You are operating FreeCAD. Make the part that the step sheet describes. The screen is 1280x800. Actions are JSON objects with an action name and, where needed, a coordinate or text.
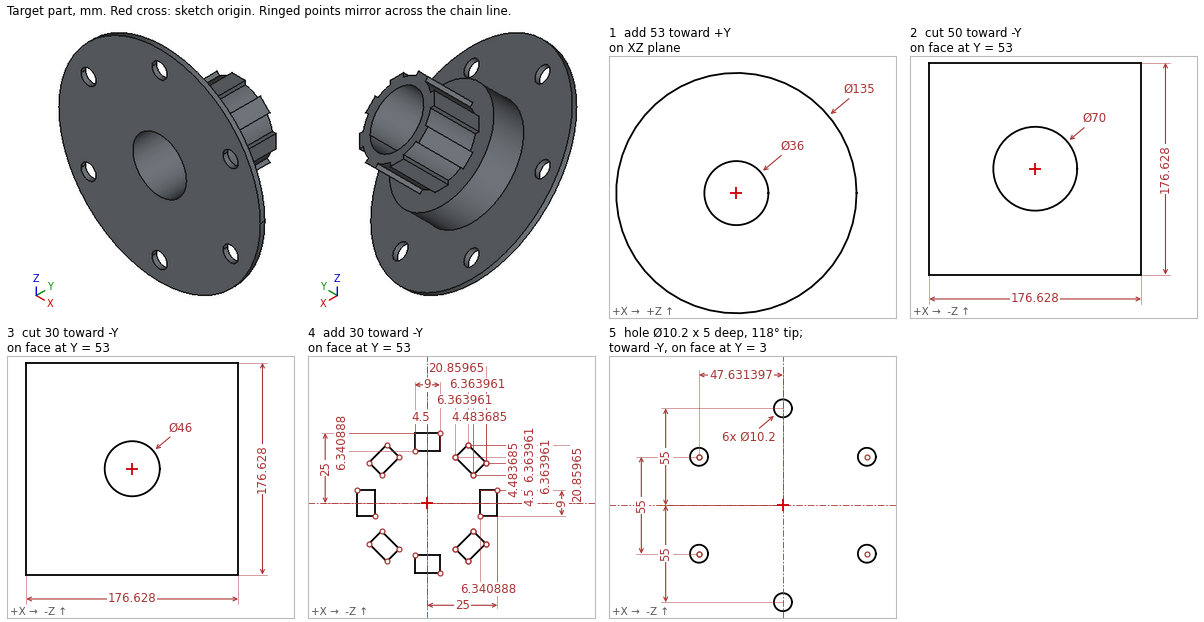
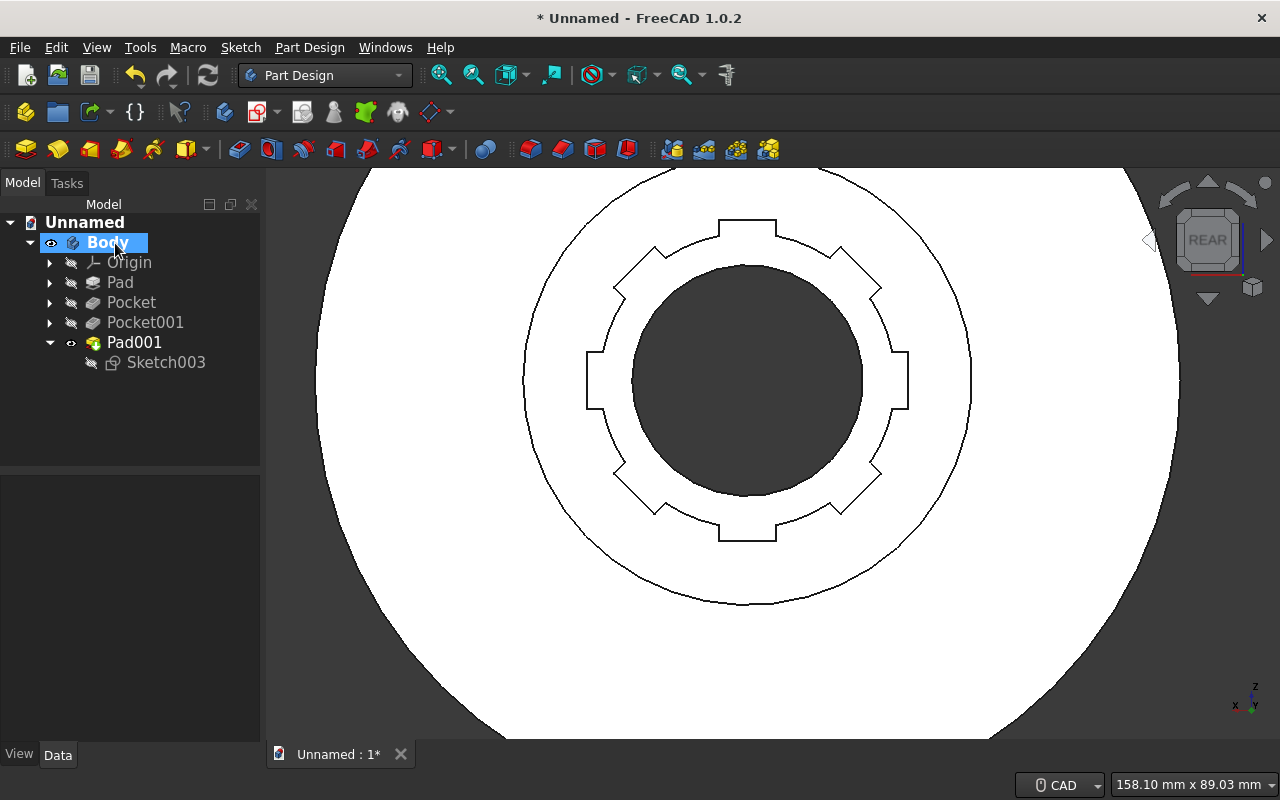
{"action": "left_click", "coordinate": [442, 76]}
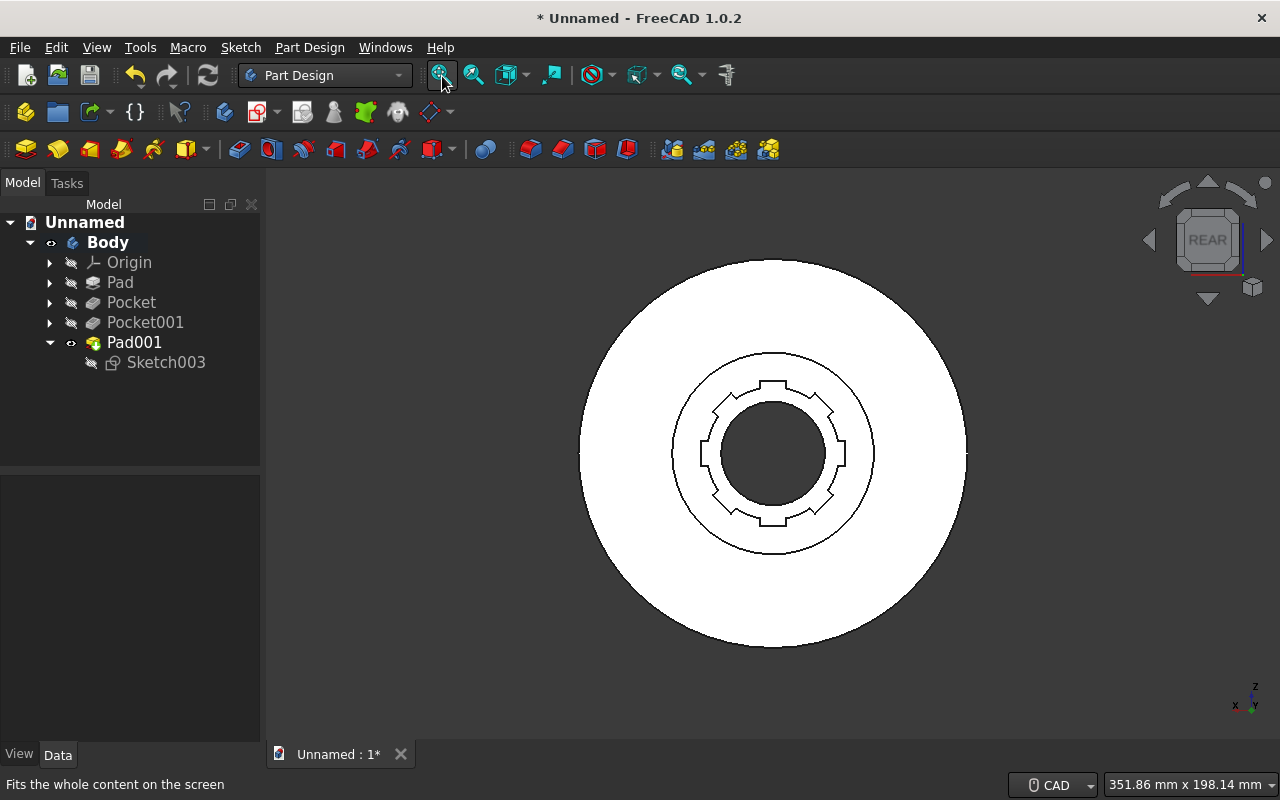
{"action": "left_click", "coordinate": [662, 341]}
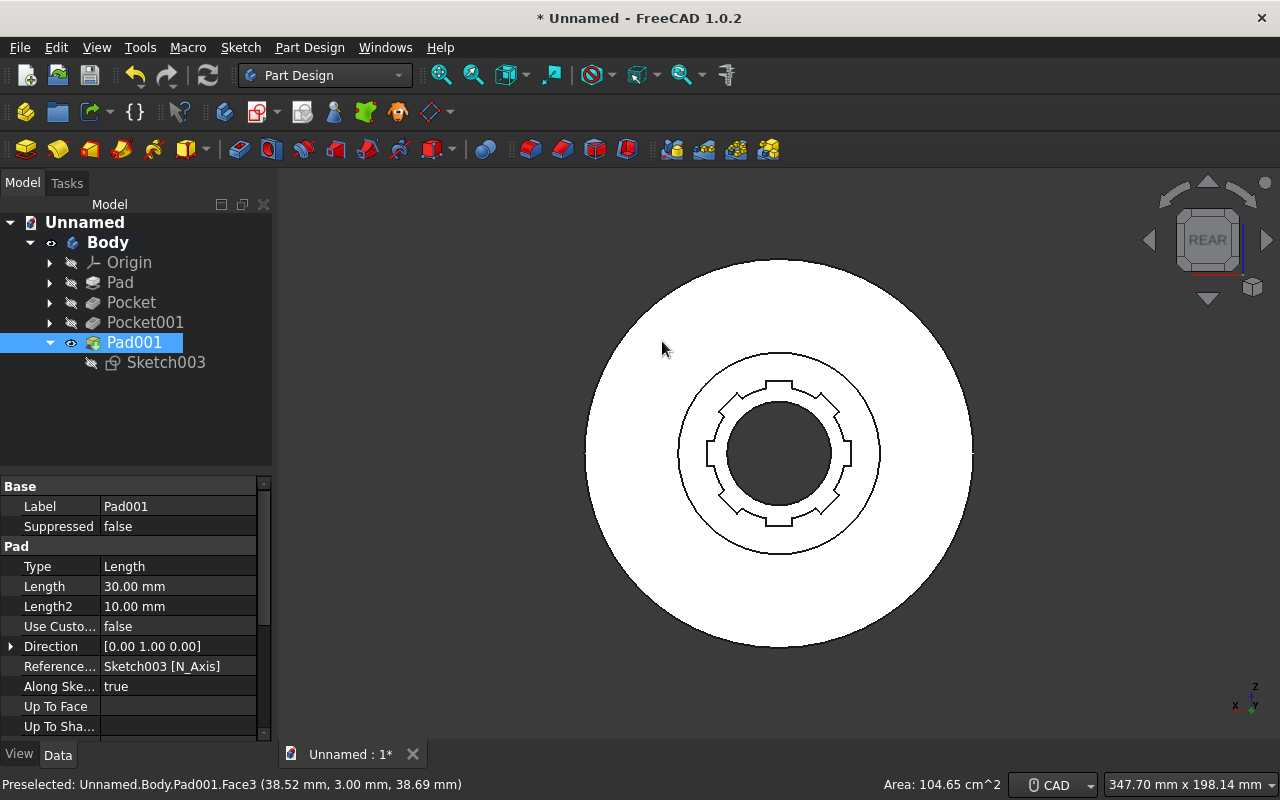
{"action": "left_click", "coordinate": [258, 112]}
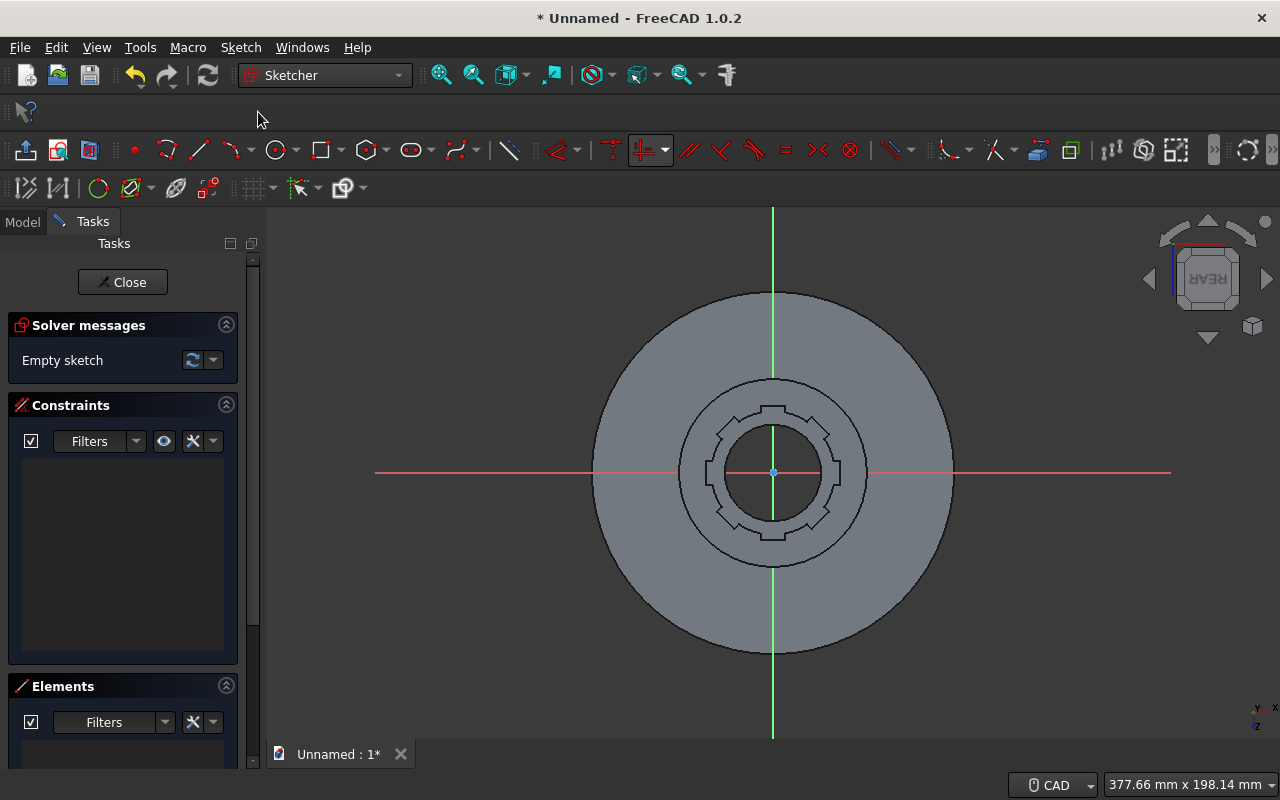
{"action": "left_click", "coordinate": [90, 150]}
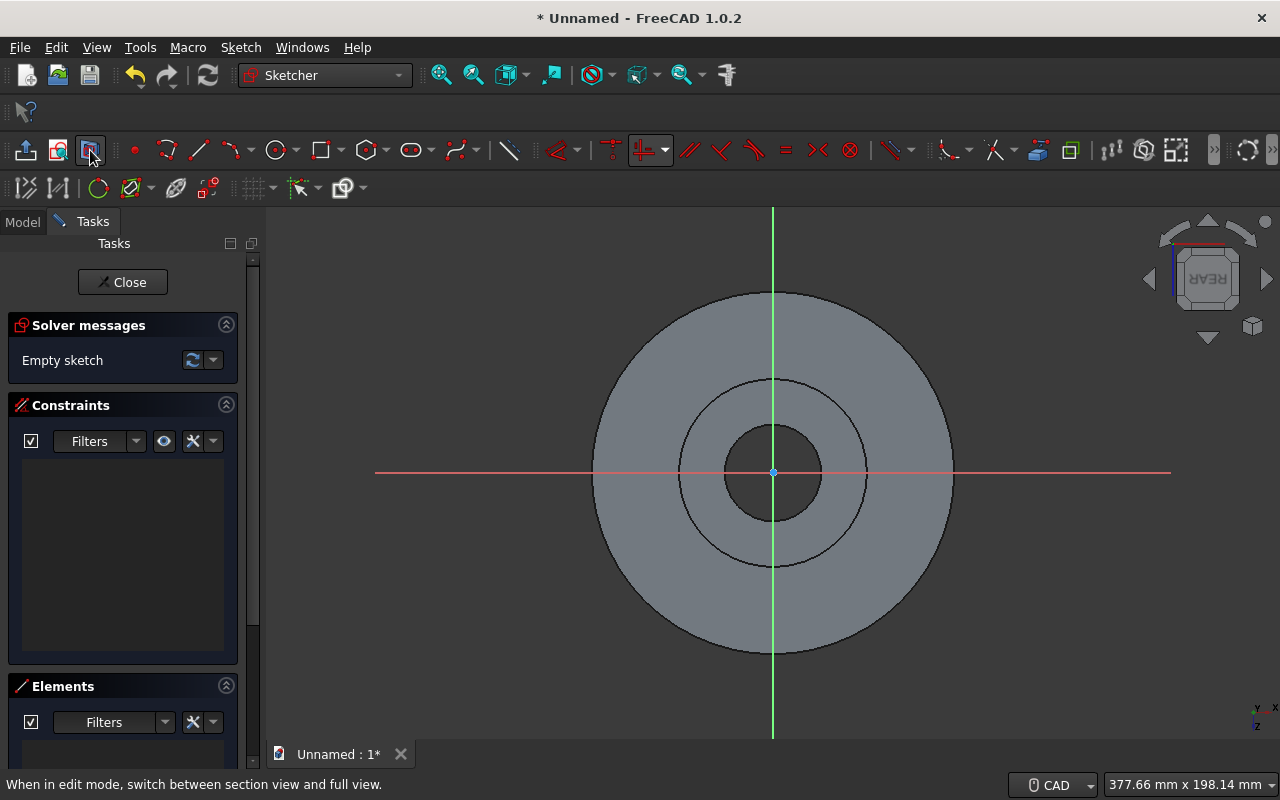
{"action": "left_click", "coordinate": [276, 150]}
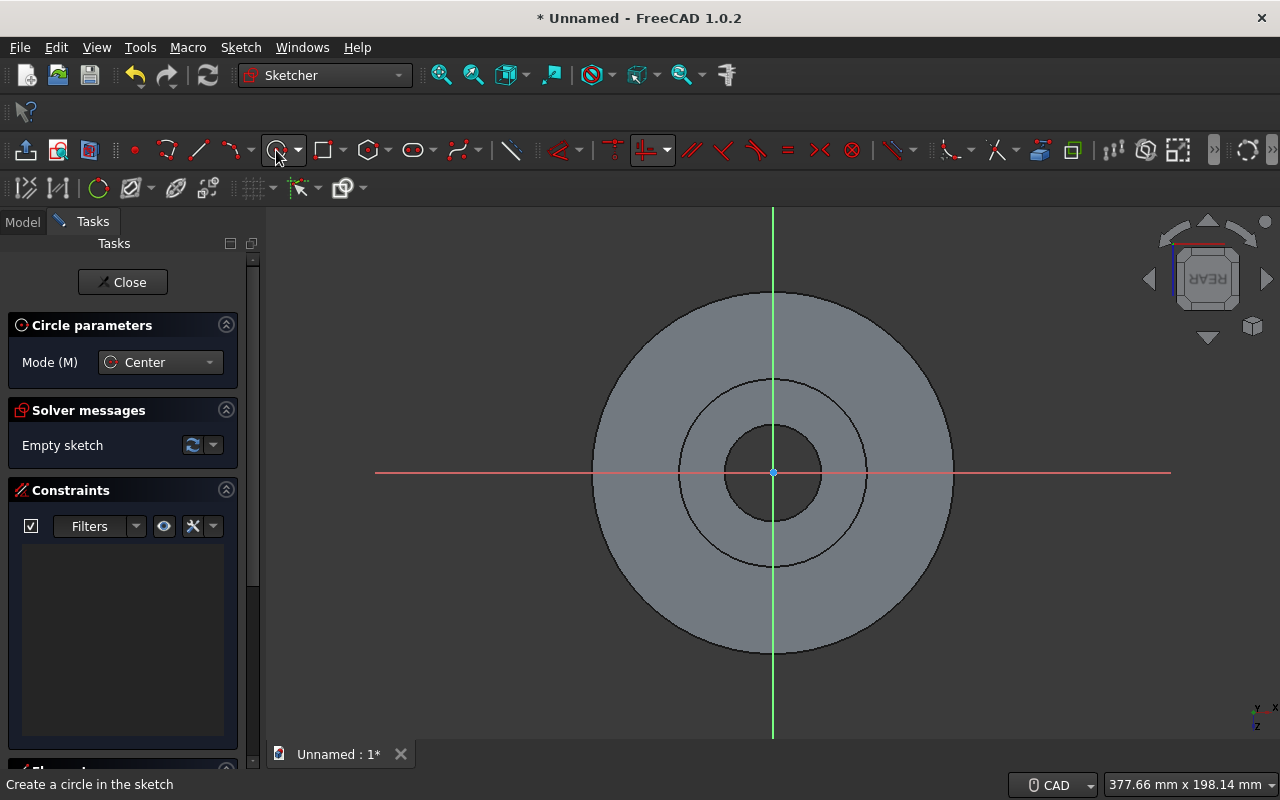
{"action": "scroll", "coordinate": [773, 325], "scroll_direction": "up", "scroll_amount": 3}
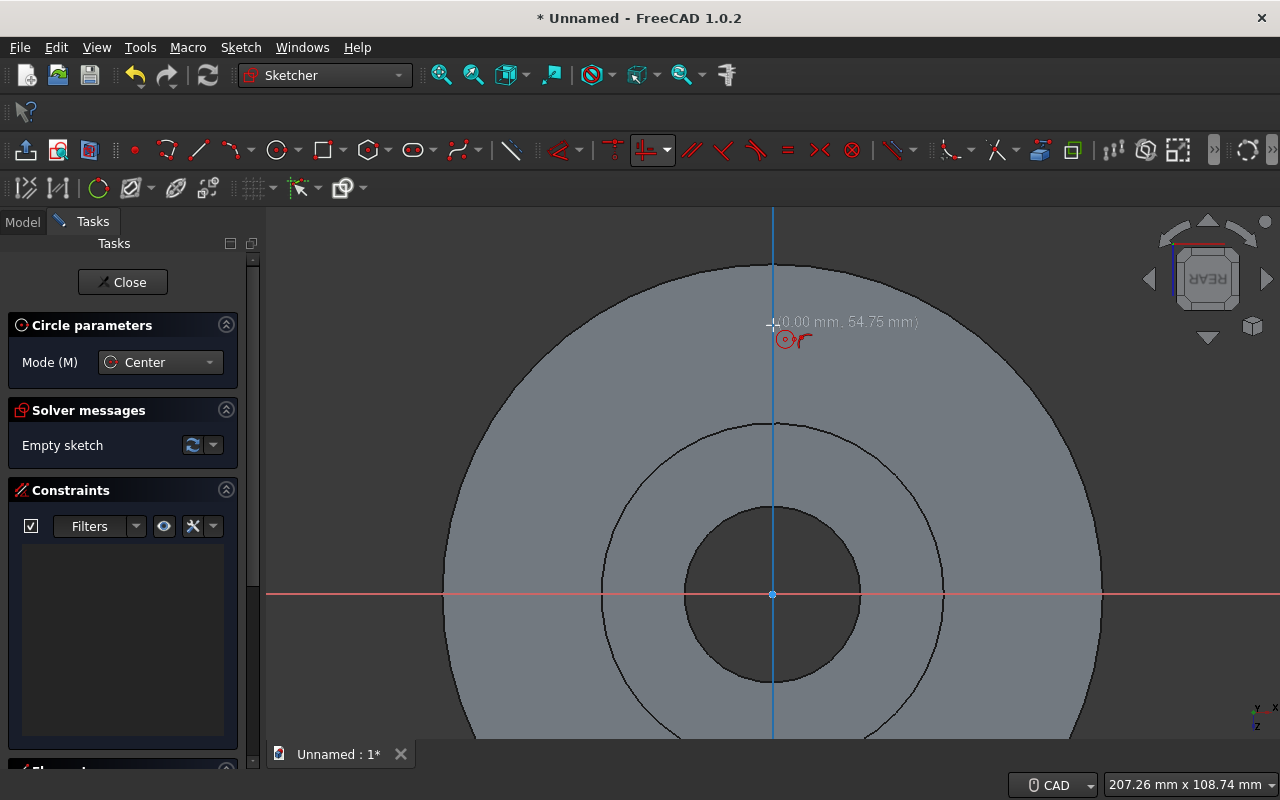
{"action": "left_click", "coordinate": [773, 325]}
{"action": "left_click", "coordinate": [790, 308]}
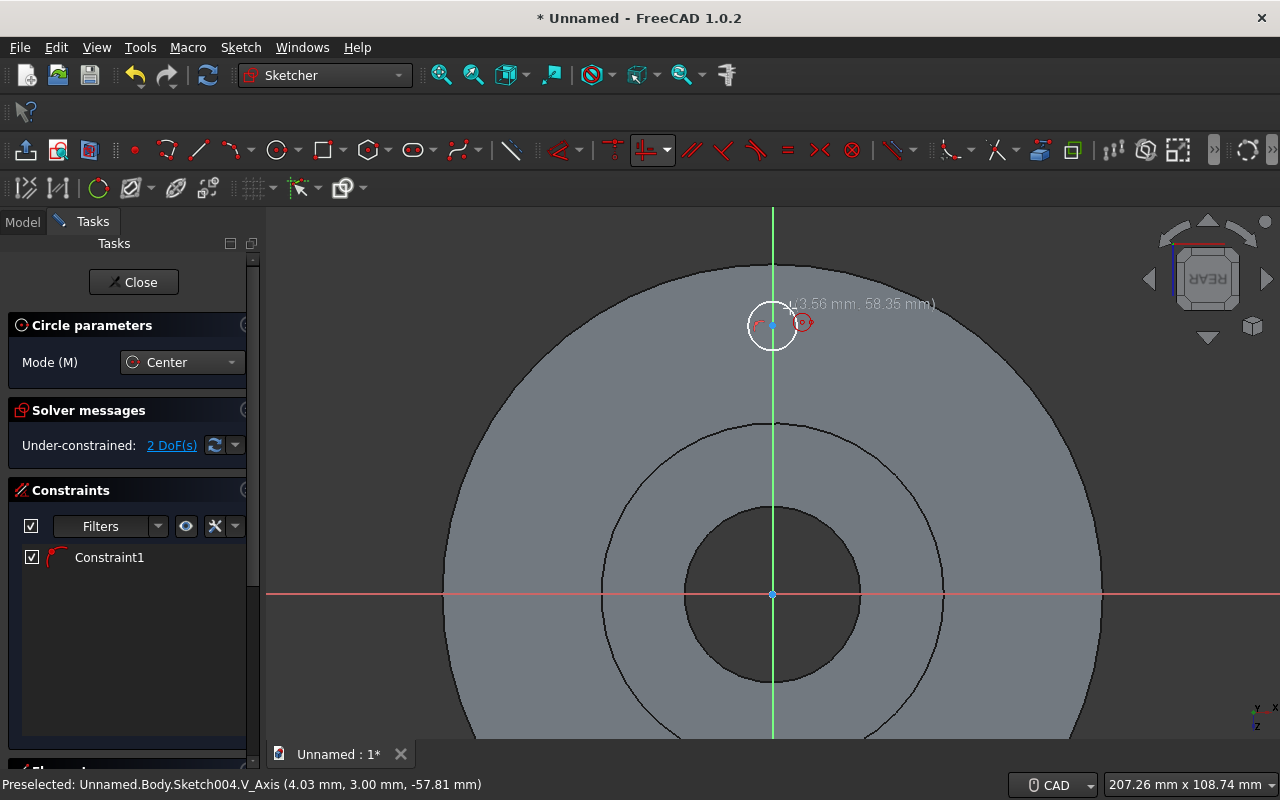
{"action": "left_click", "coordinate": [540, 460]}
{"action": "left_click", "coordinate": [557, 442]}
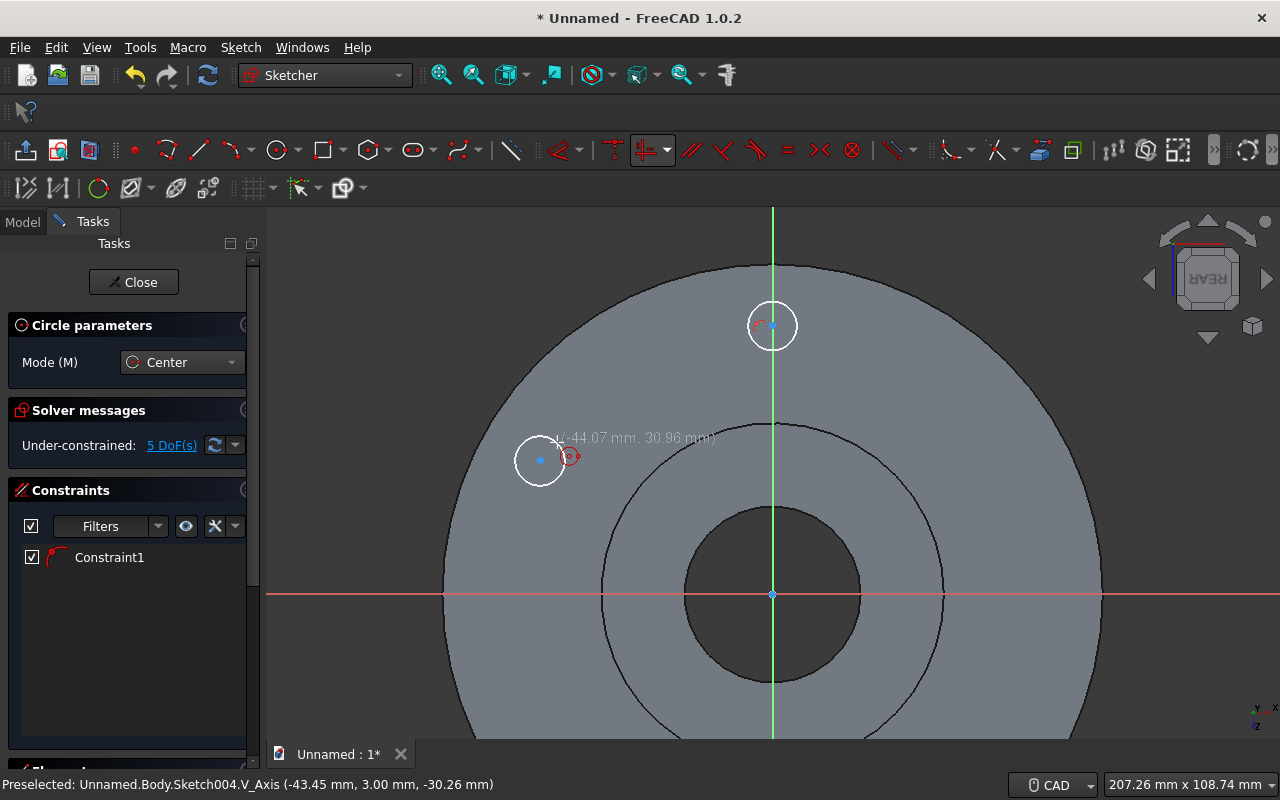
{"action": "scroll", "coordinate": [622, 325], "scroll_direction": "down", "scroll_amount": 3}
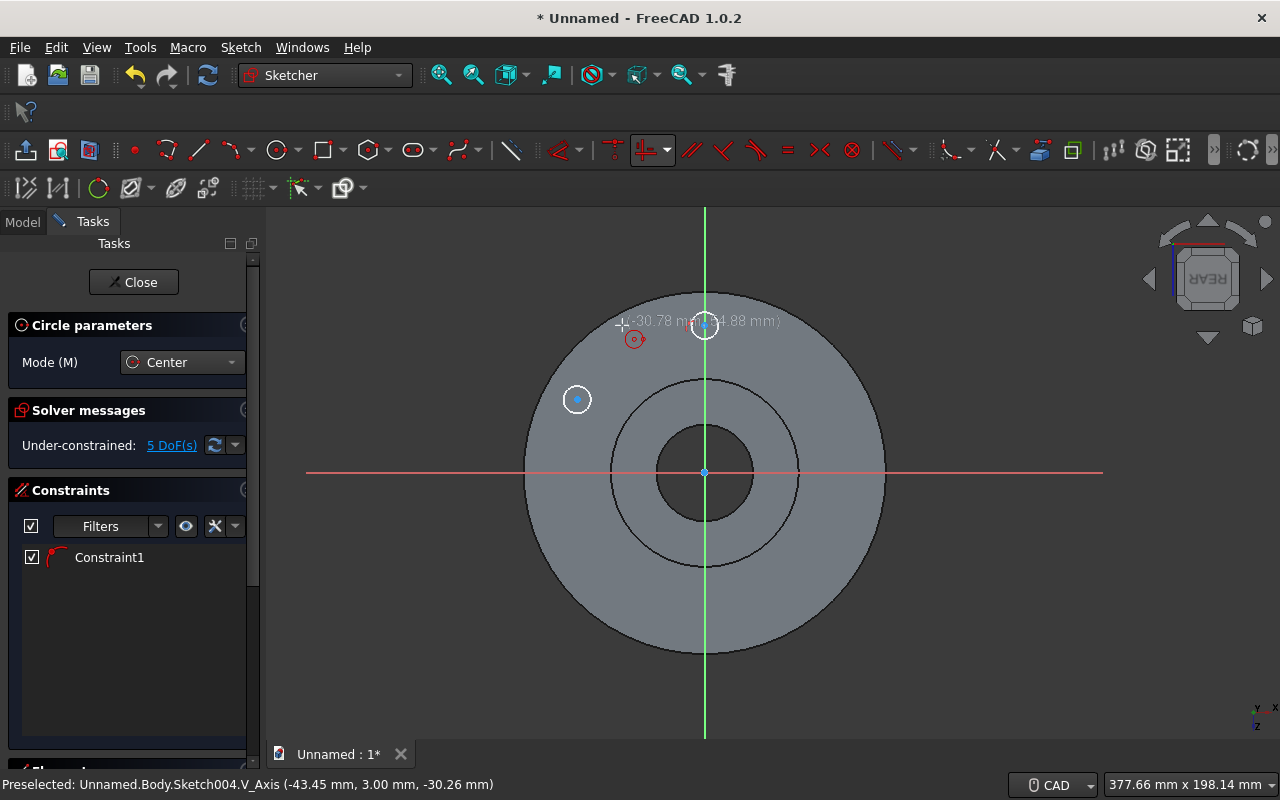
{"action": "scroll", "coordinate": [577, 547], "scroll_direction": "up", "scroll_amount": 3}